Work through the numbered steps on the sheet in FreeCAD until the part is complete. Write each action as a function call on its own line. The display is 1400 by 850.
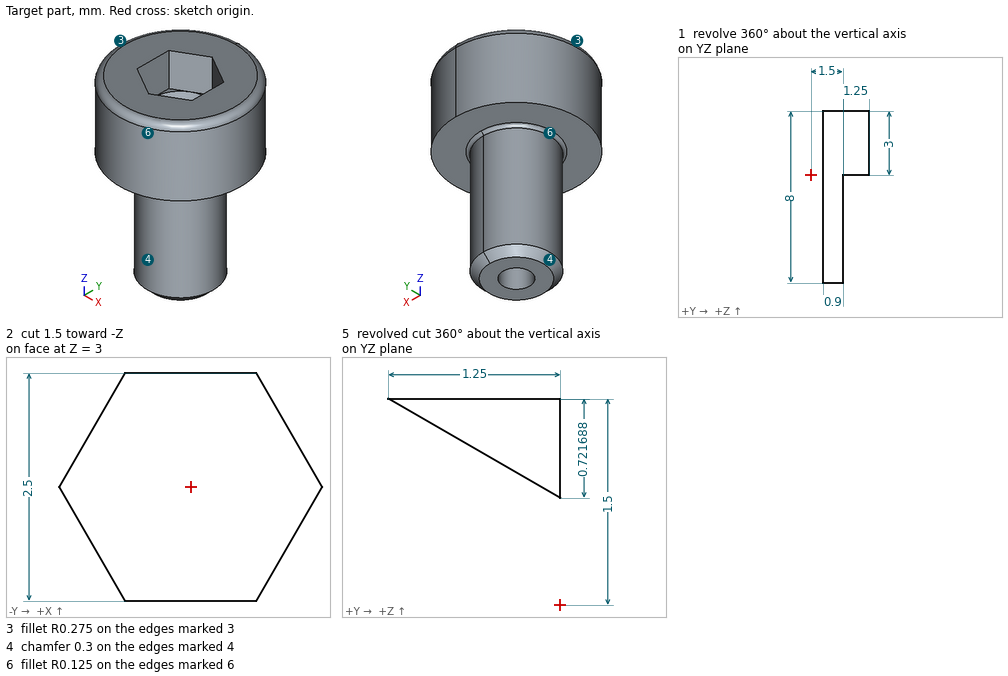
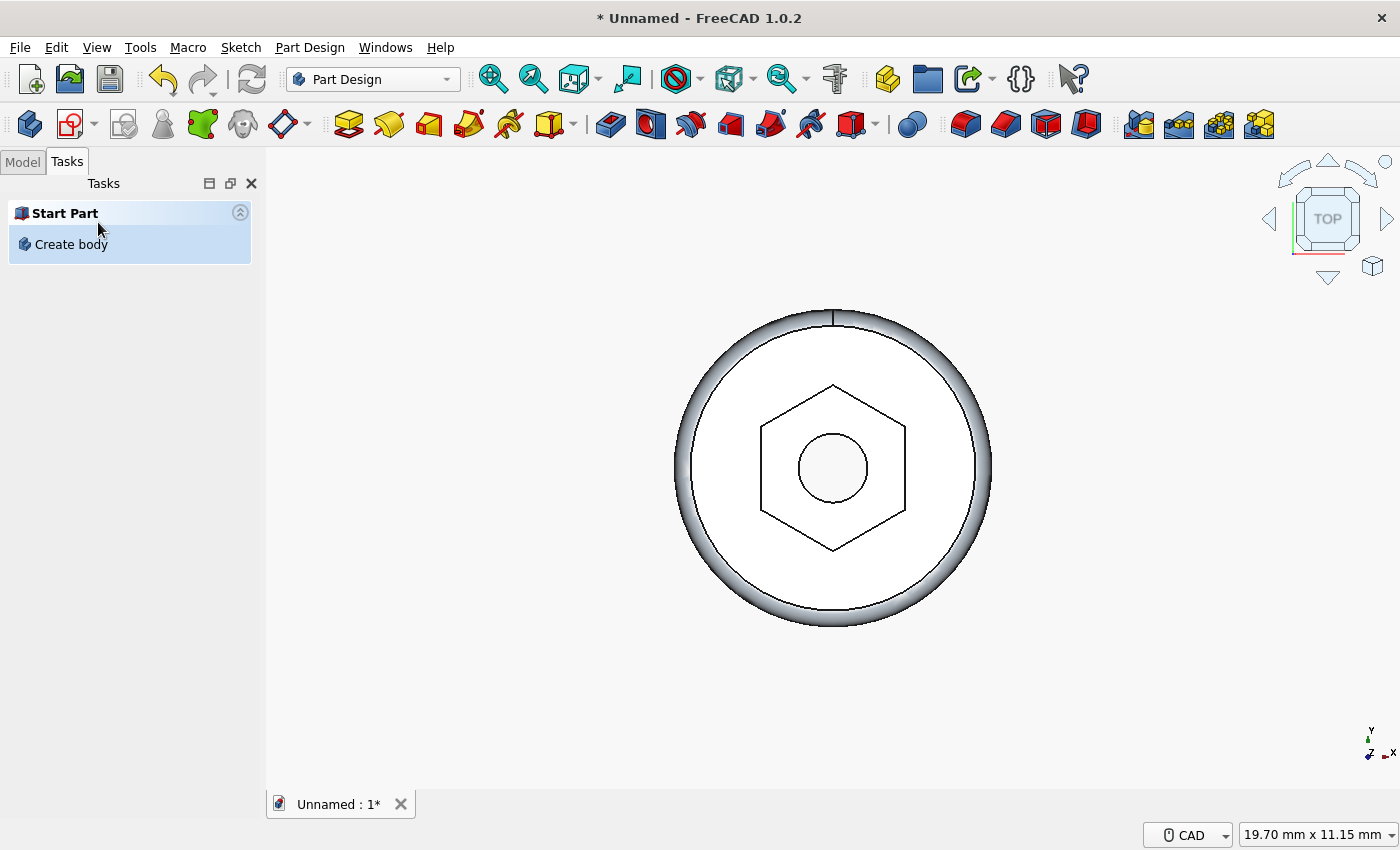
key(1)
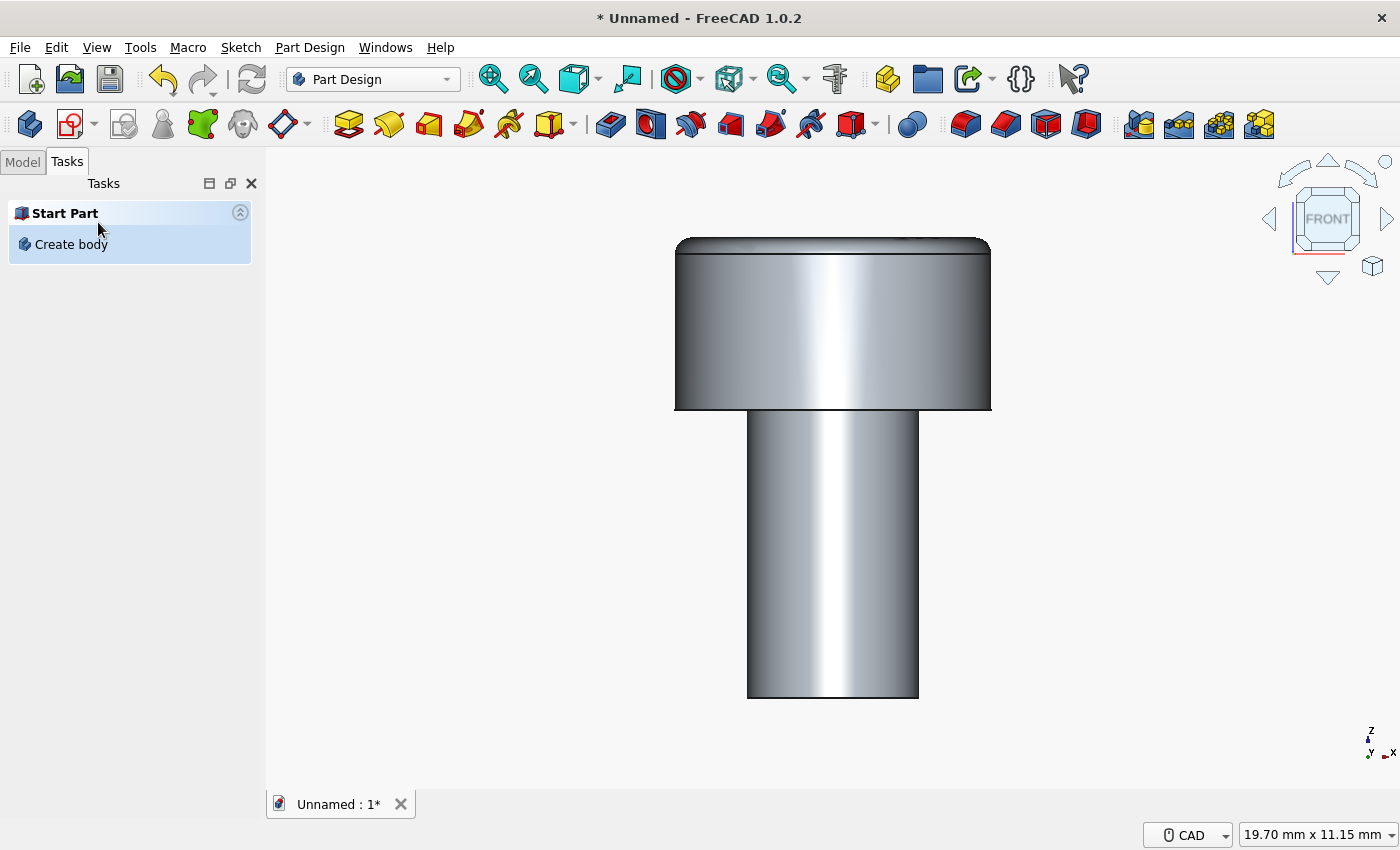
click(833, 697)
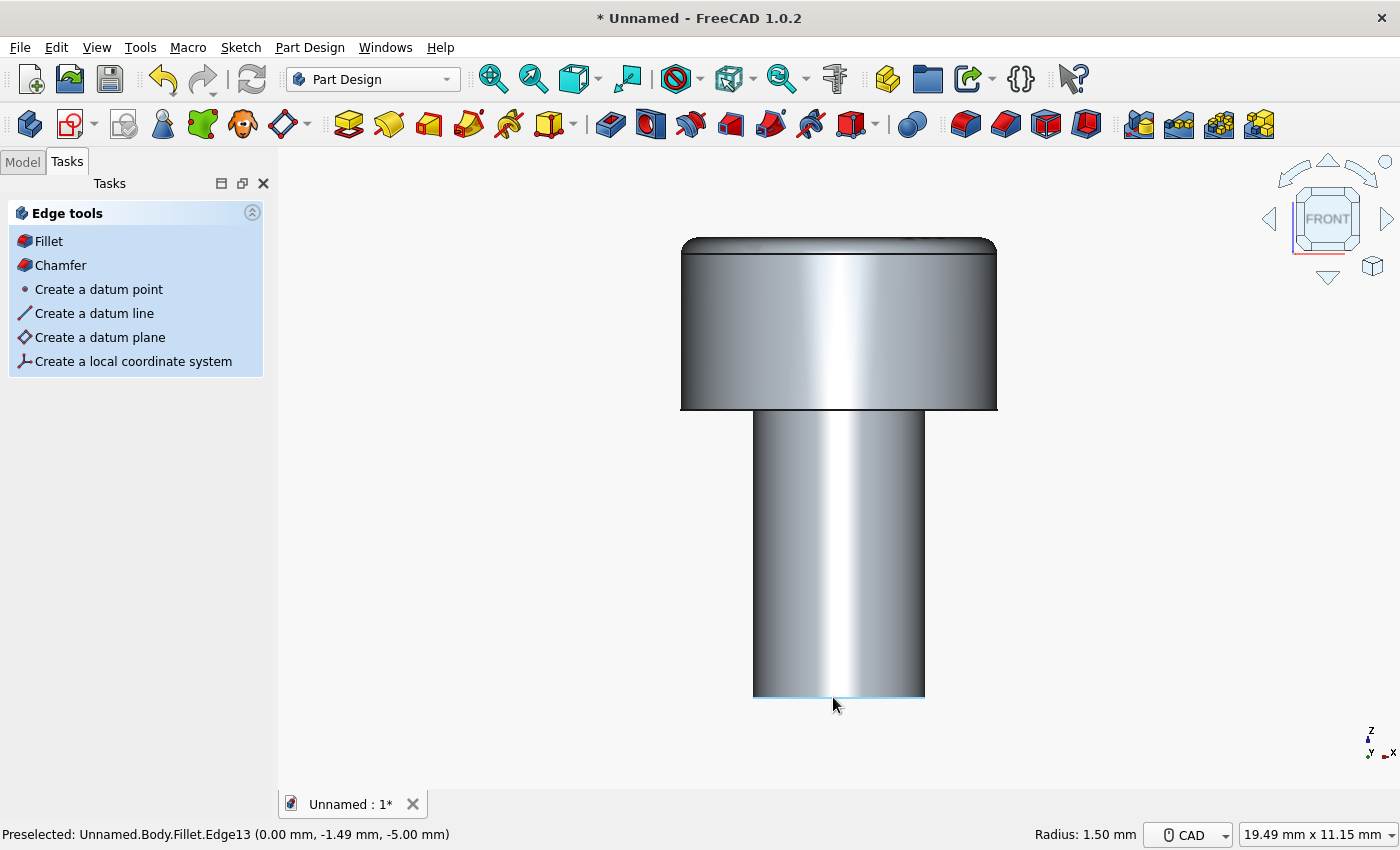
click(1006, 124)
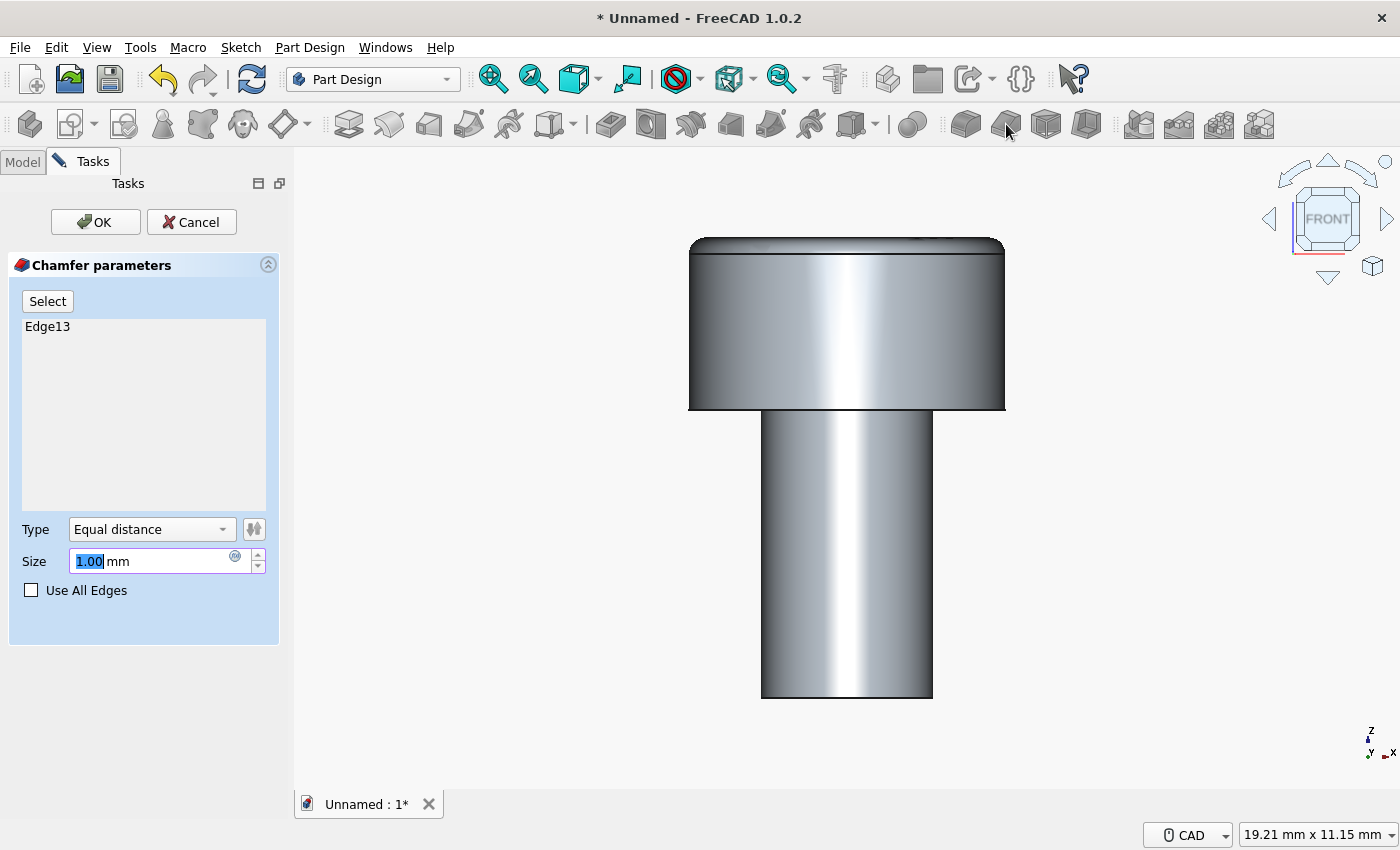
text(0.3)
key(Tab)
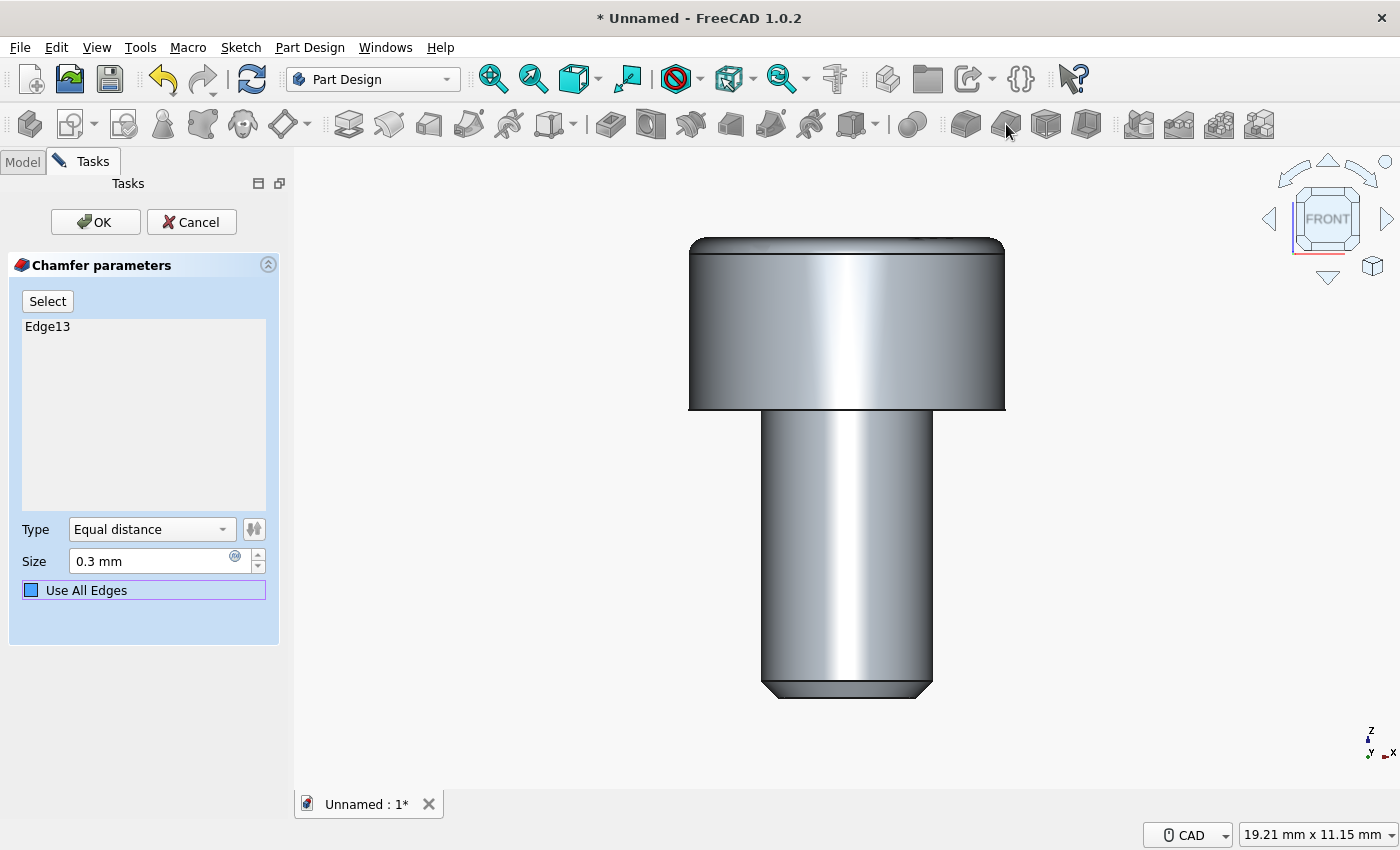
click(96, 222)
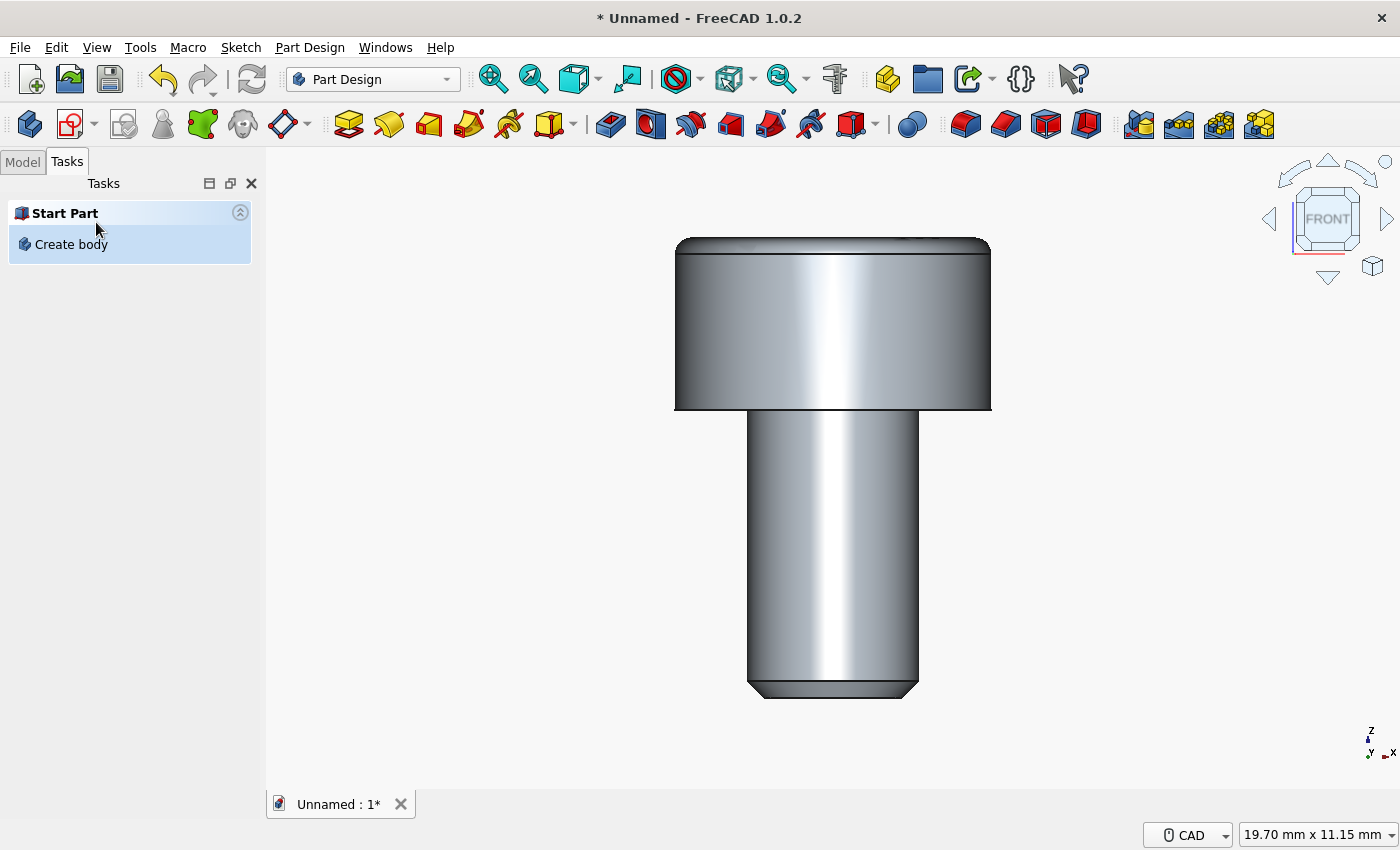
click(70, 124)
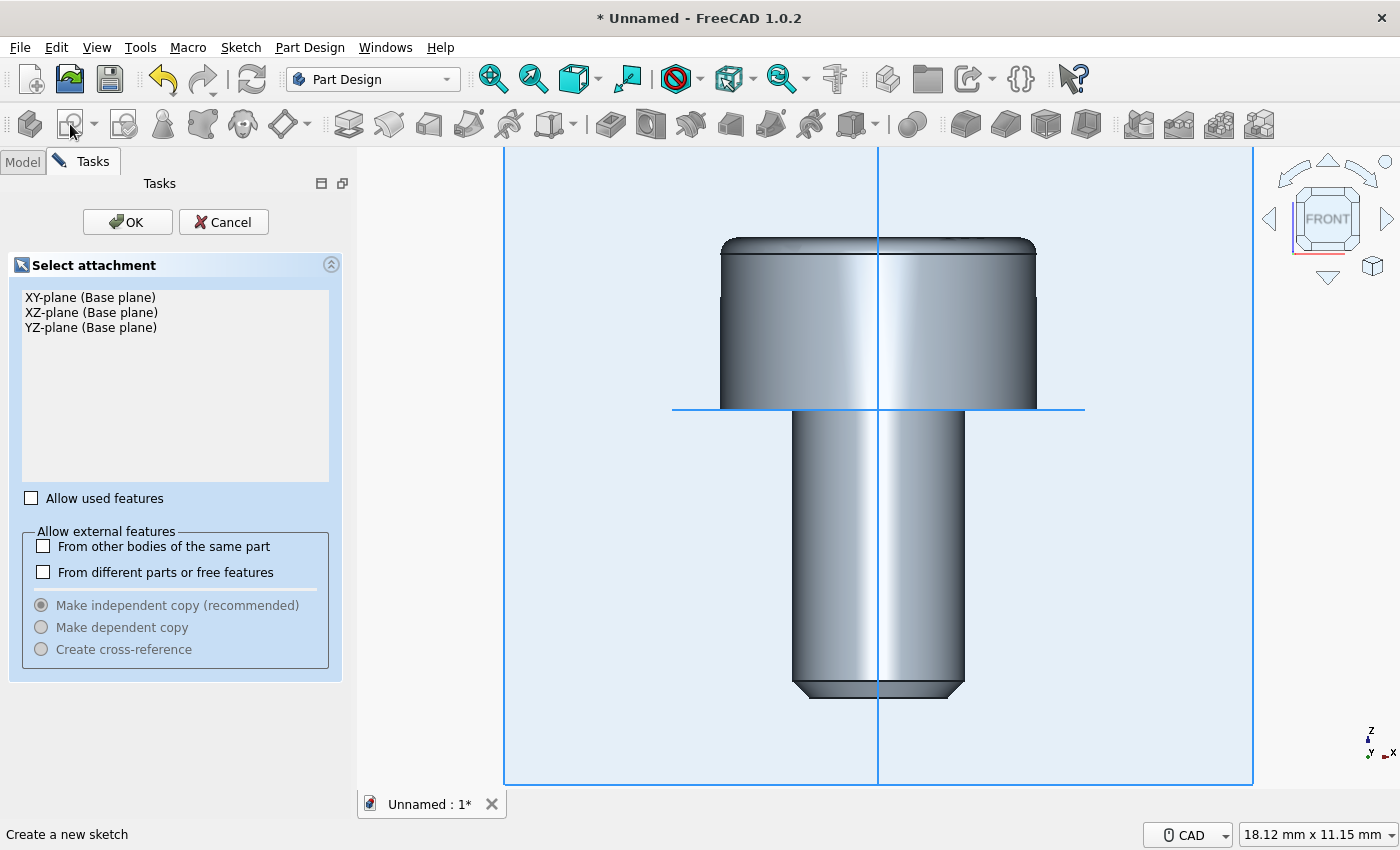
click(82, 328)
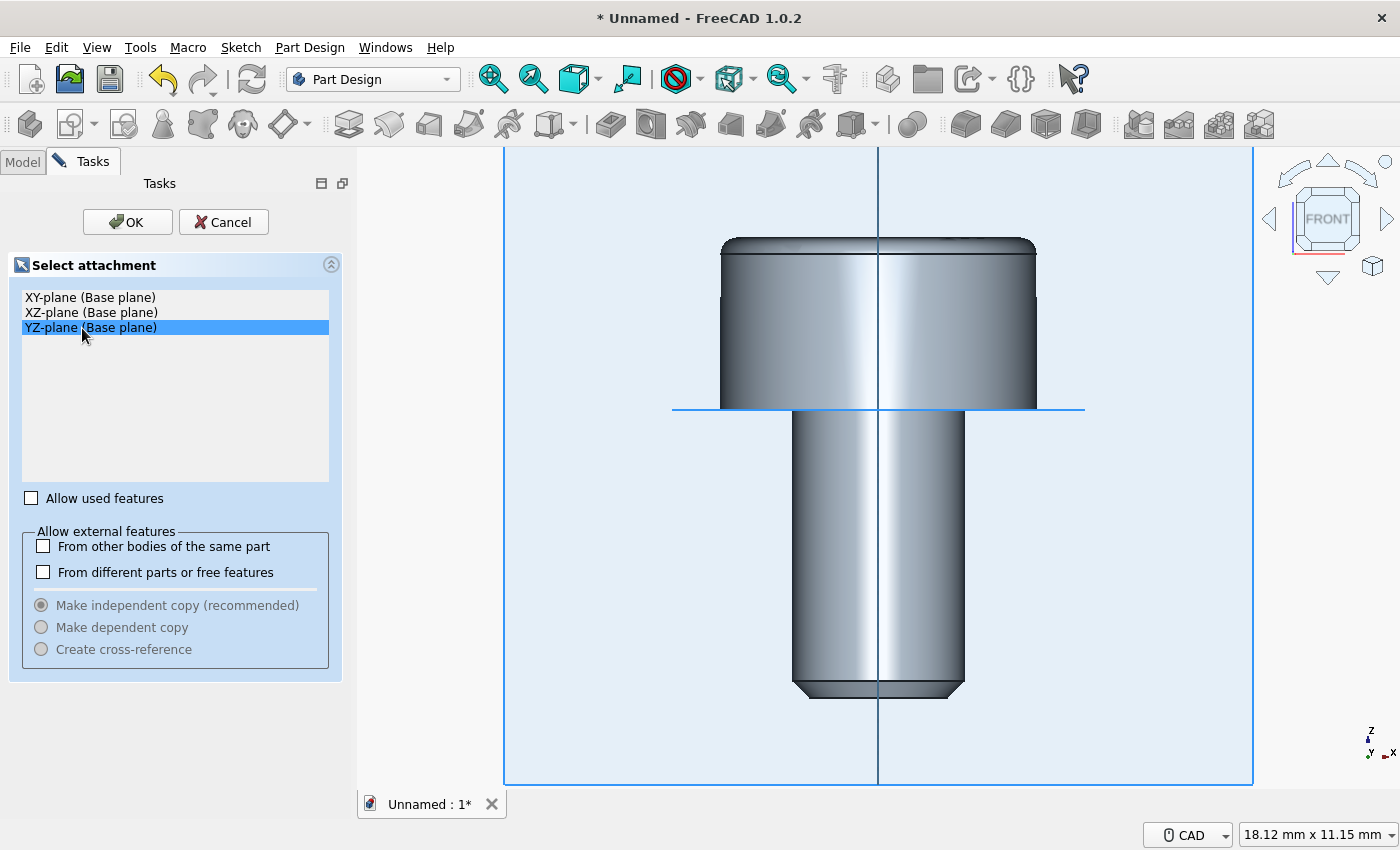
click(128, 222)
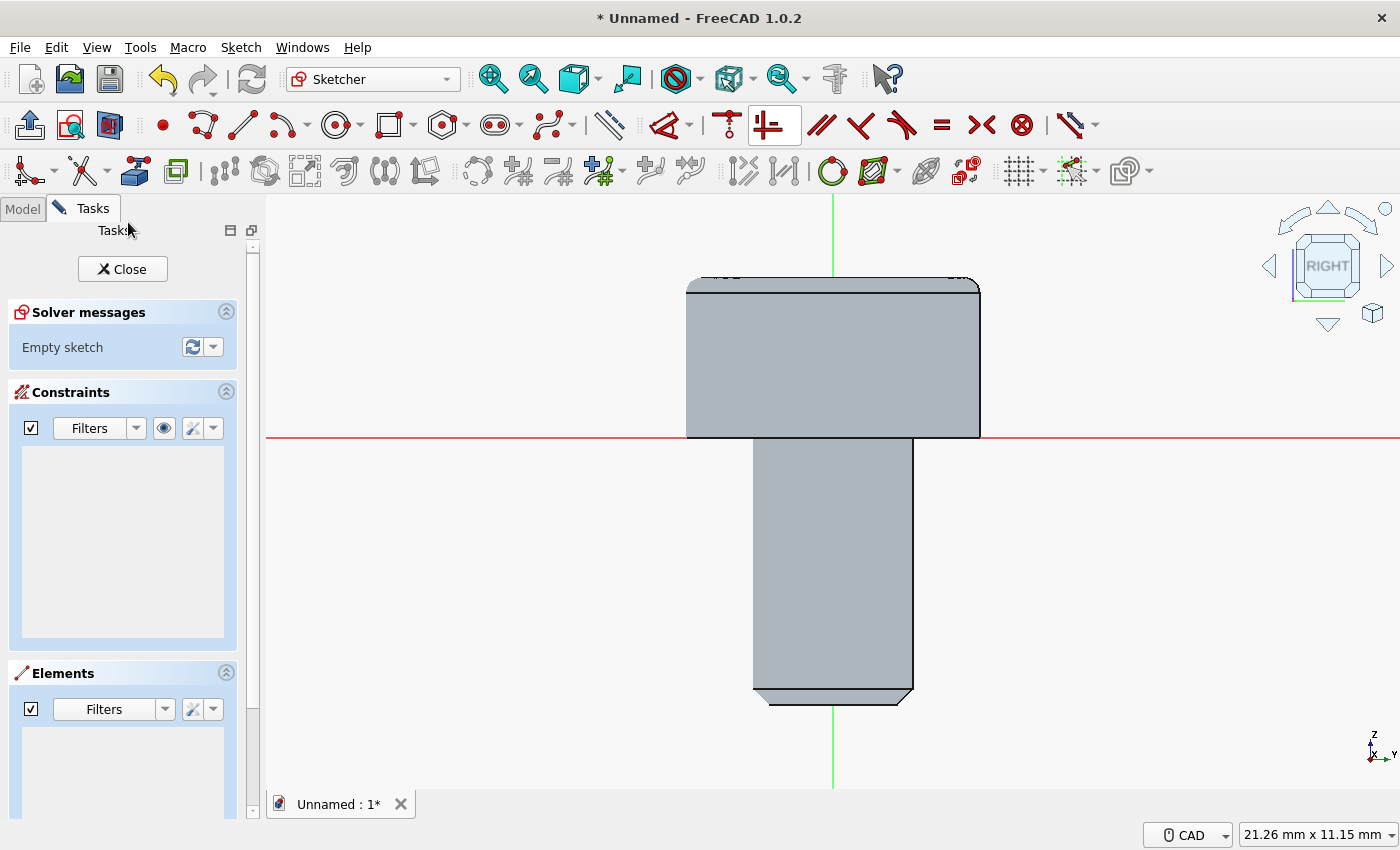
click(110, 126)